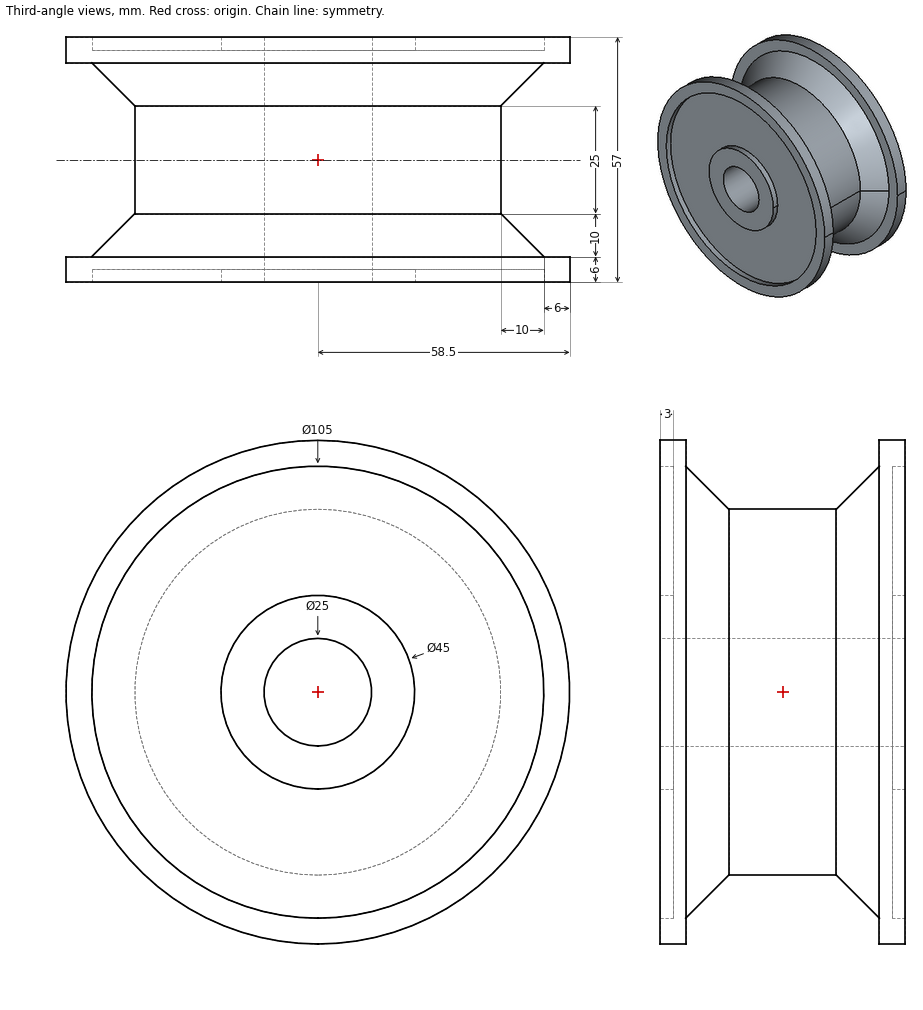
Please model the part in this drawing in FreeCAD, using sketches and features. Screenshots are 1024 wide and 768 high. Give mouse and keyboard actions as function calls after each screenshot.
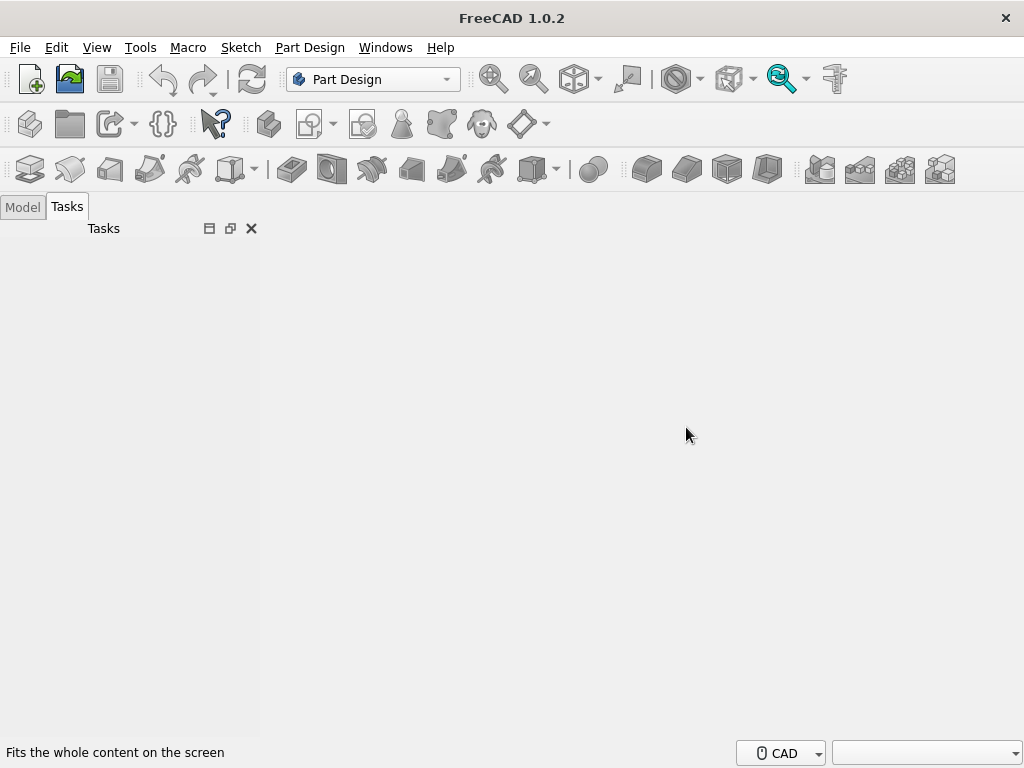
click(30, 80)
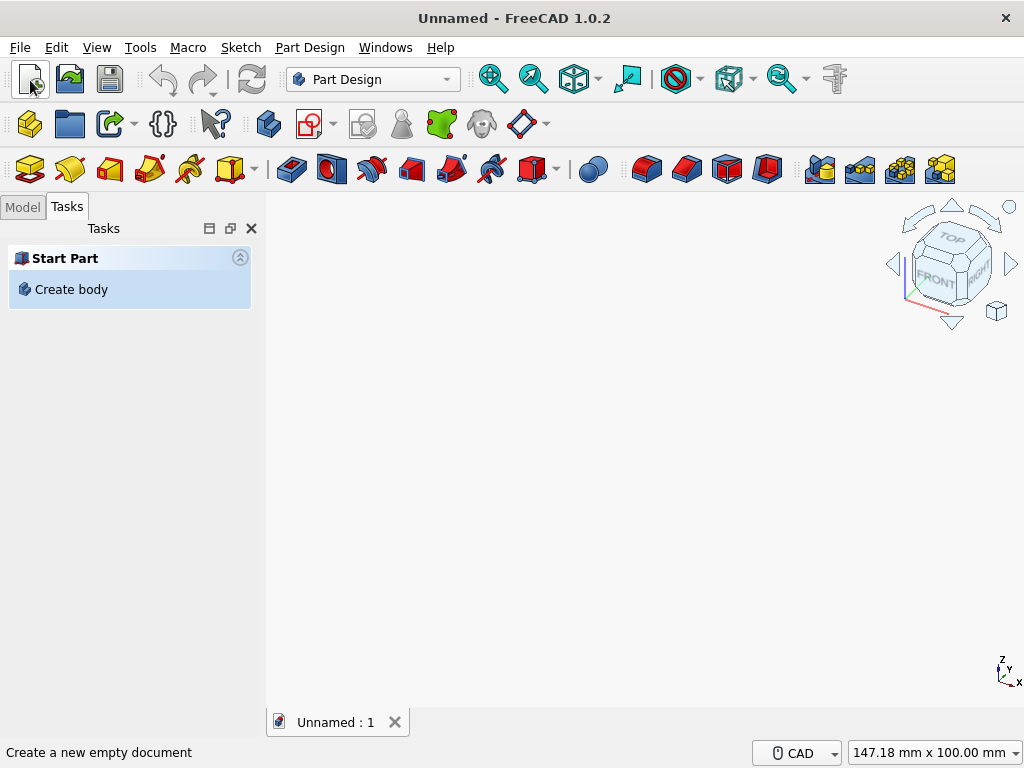
click(310, 124)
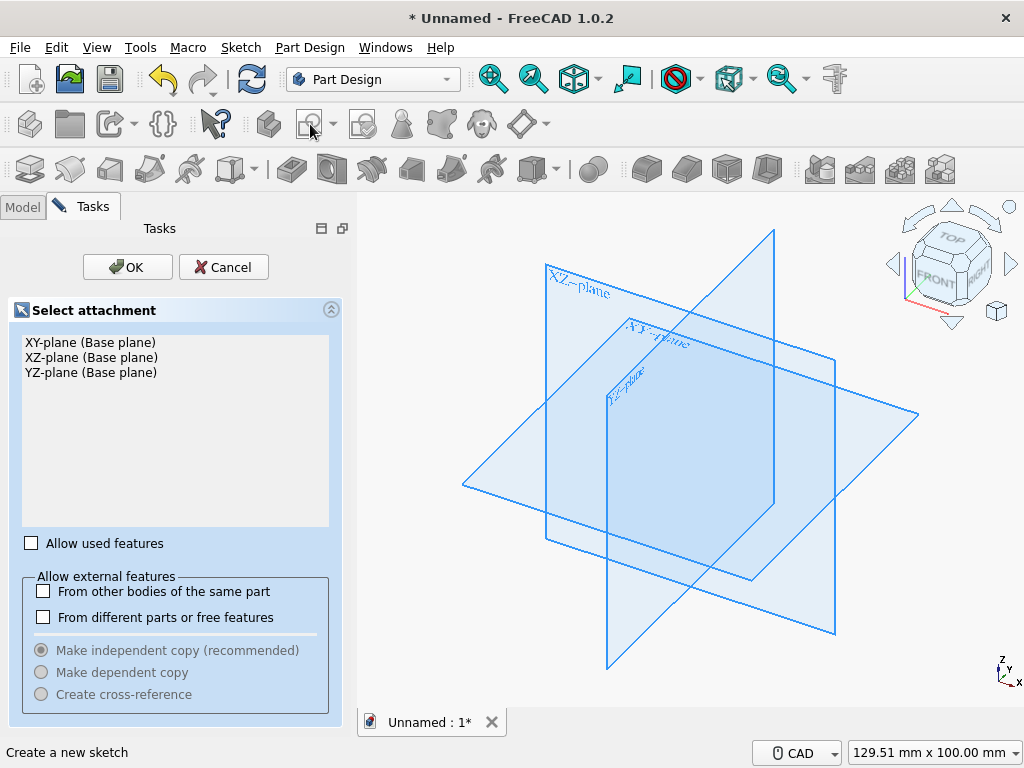
click(82, 342)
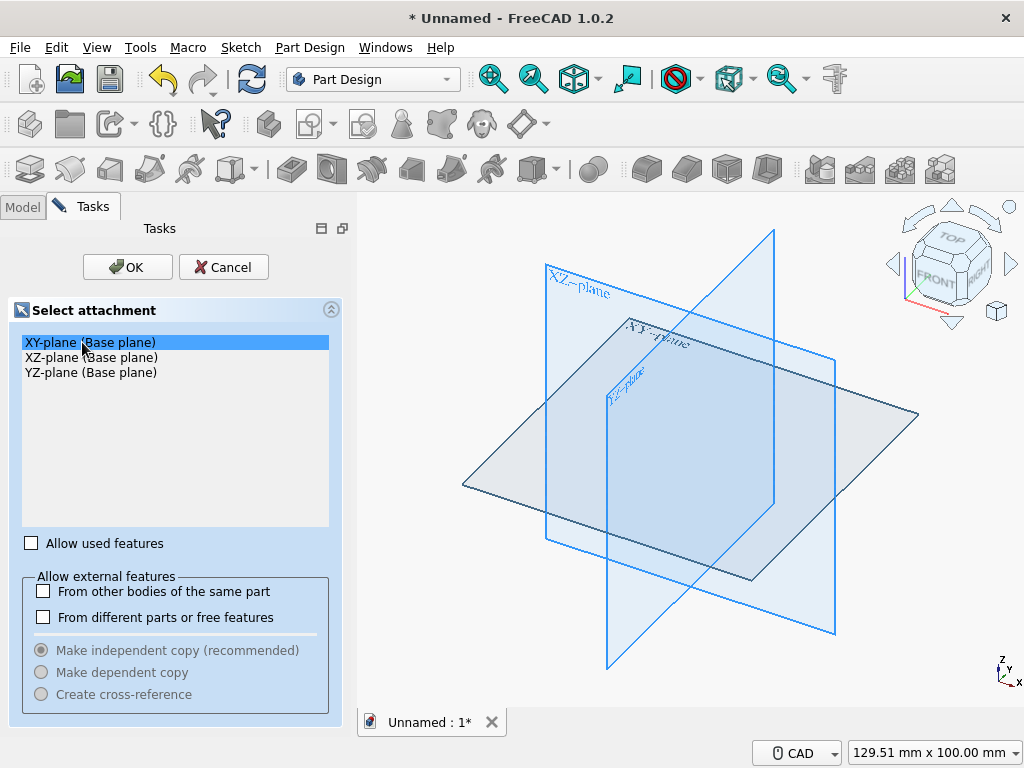
click(128, 267)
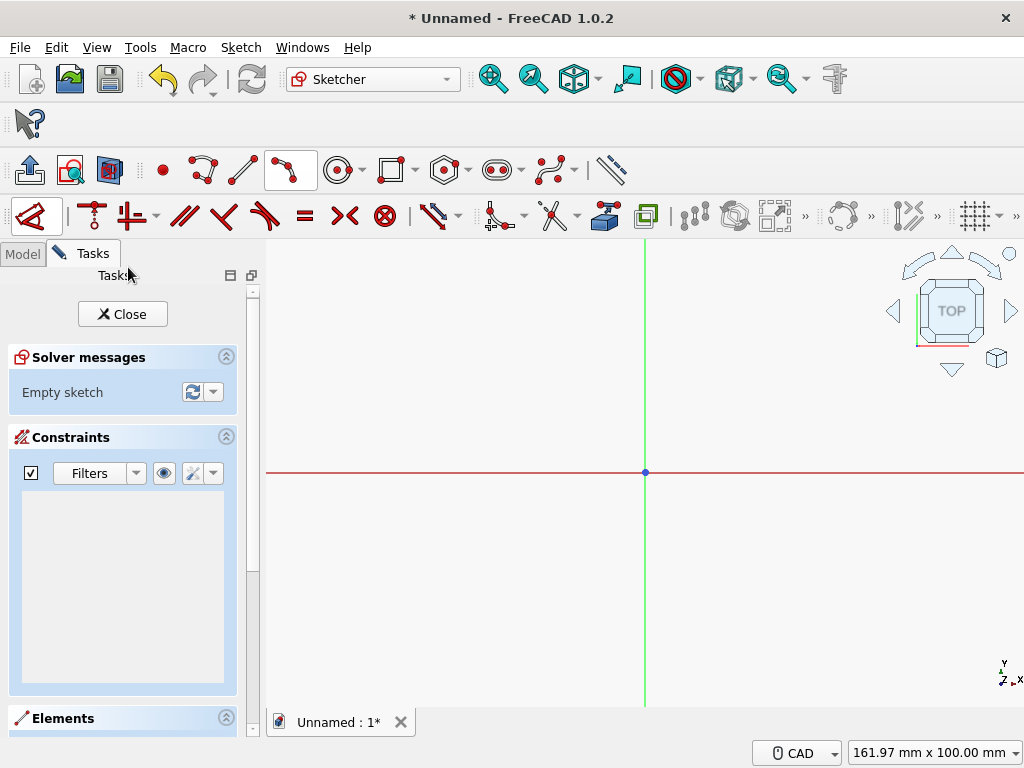
scroll(294, 473, down, 1)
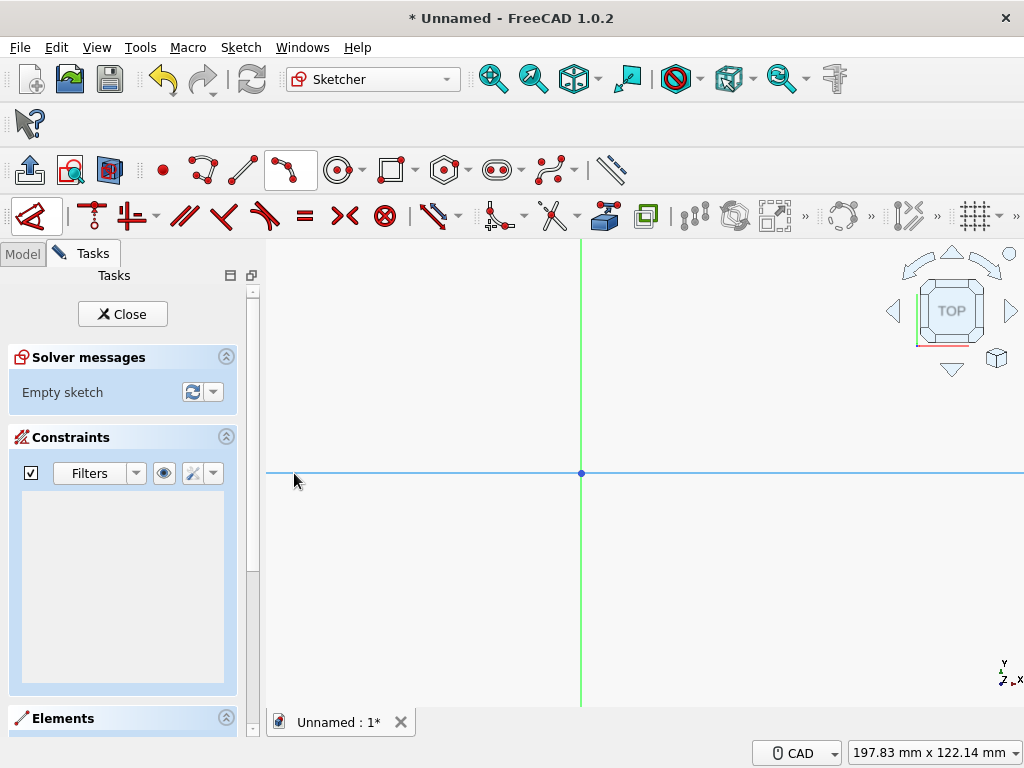
click(204, 170)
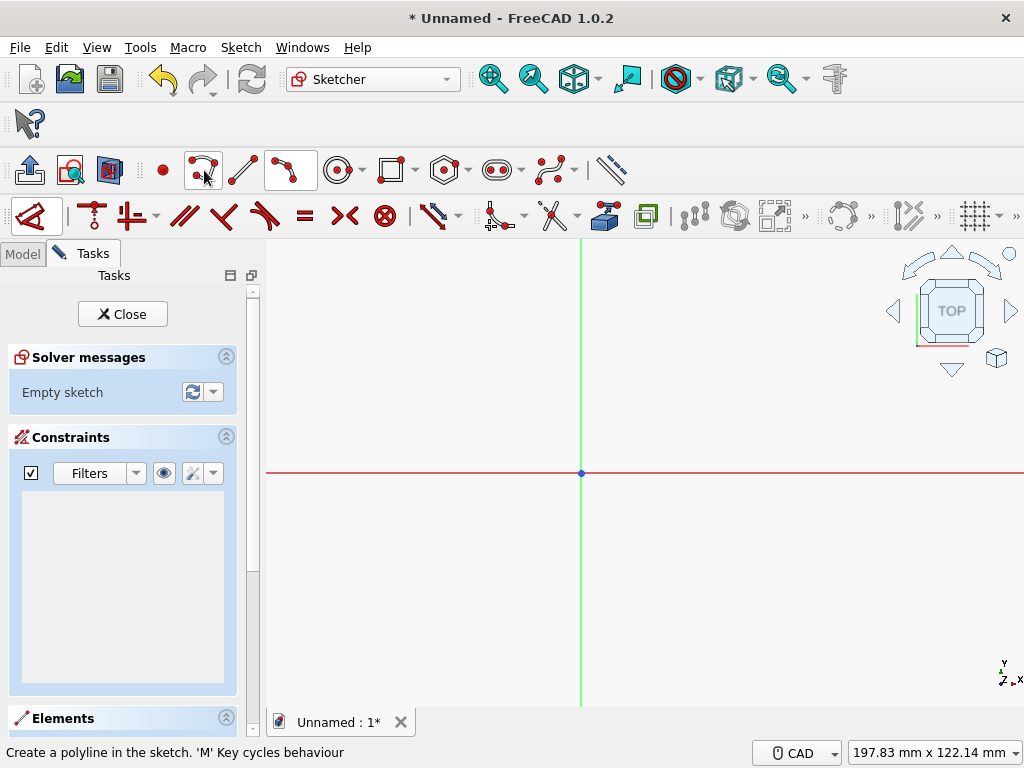
click(581, 364)
click(590, 582)
click(806, 582)
click(806, 559)
click(783, 559)
click(744, 521)
click(744, 425)
click(783, 387)
click(806, 387)
click(806, 364)
click(581, 365)
key(Escape)
key(Escape)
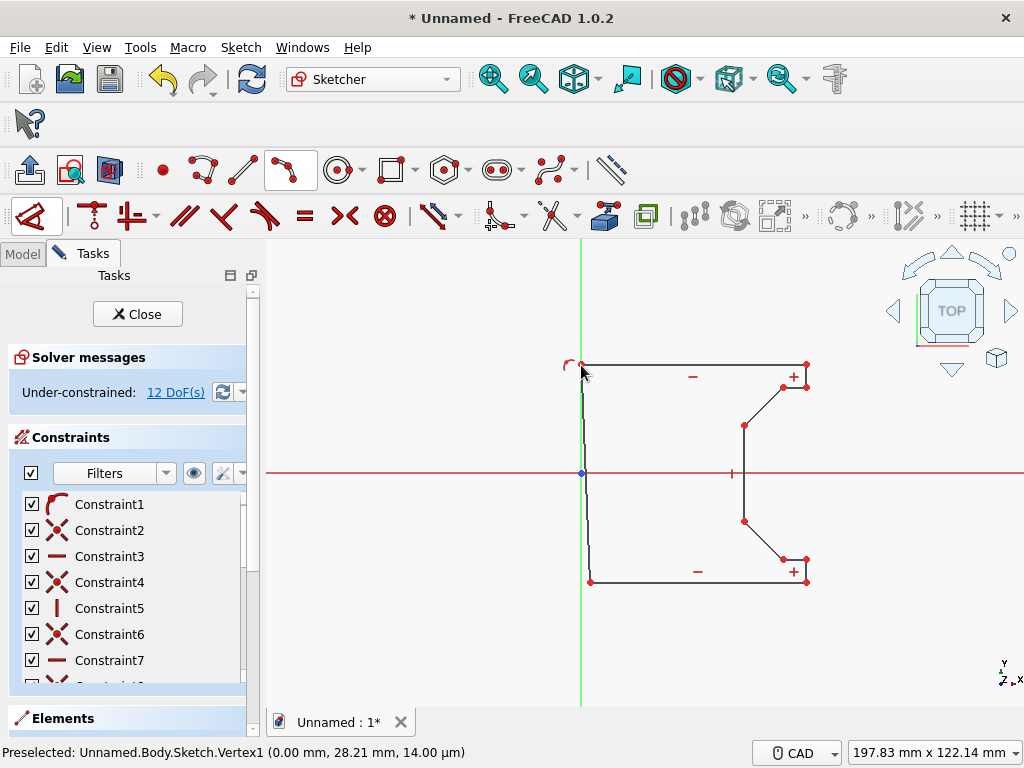
click(584, 430)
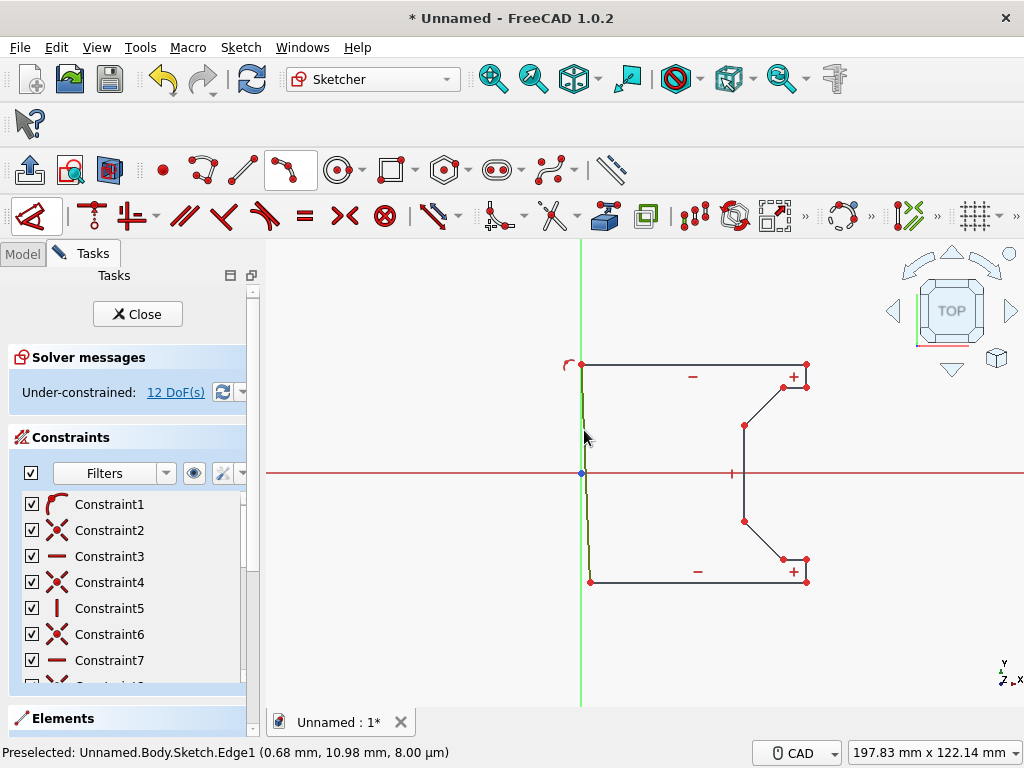
key(v)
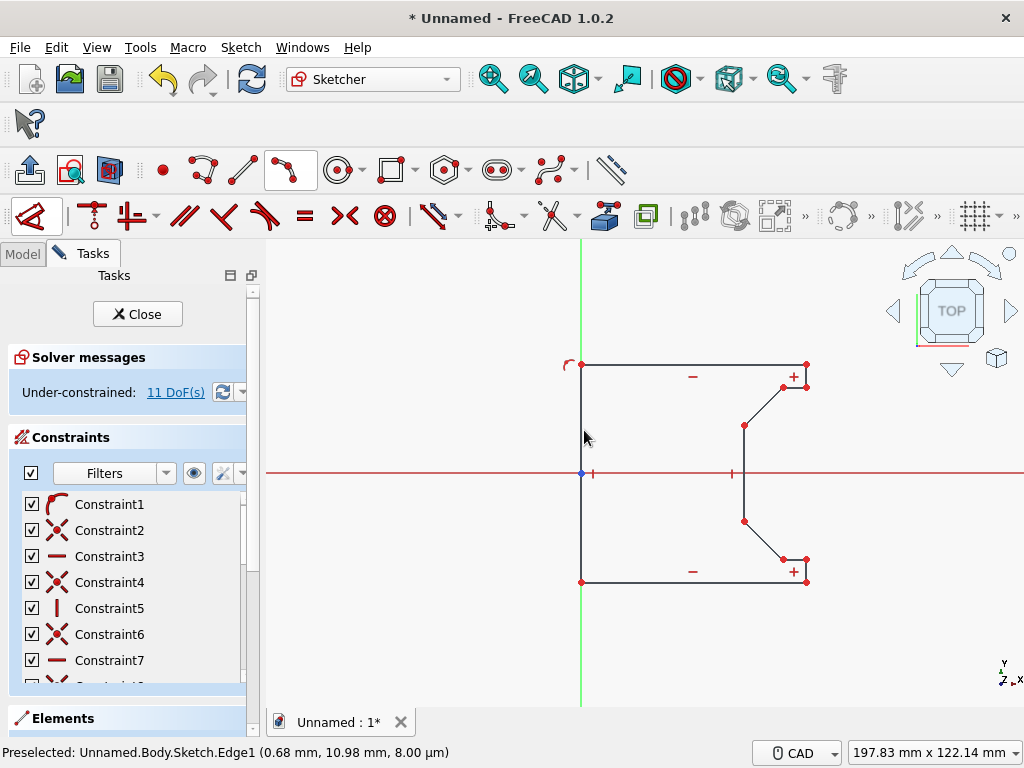
click(783, 560)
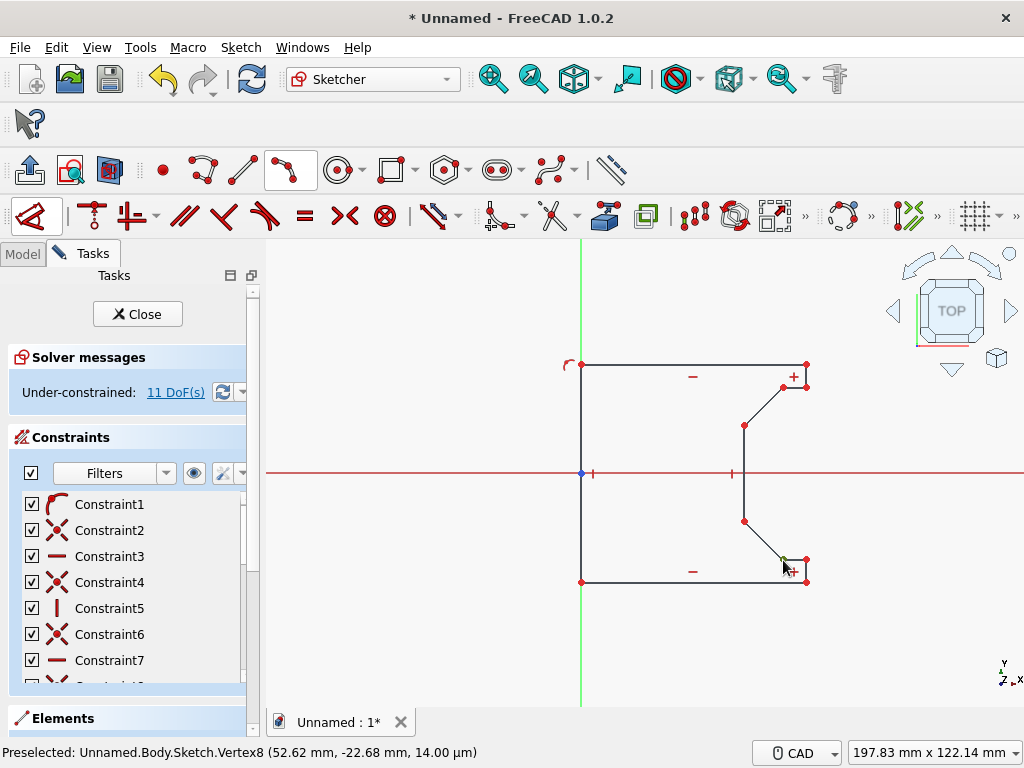
click(783, 388)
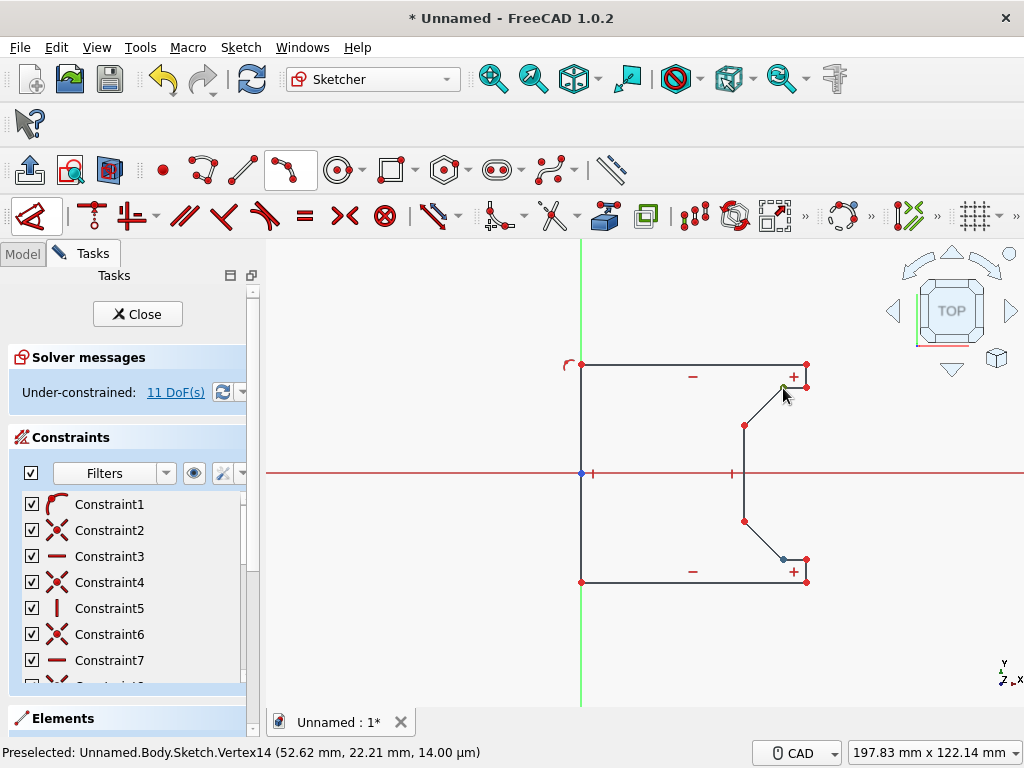
click(334, 473)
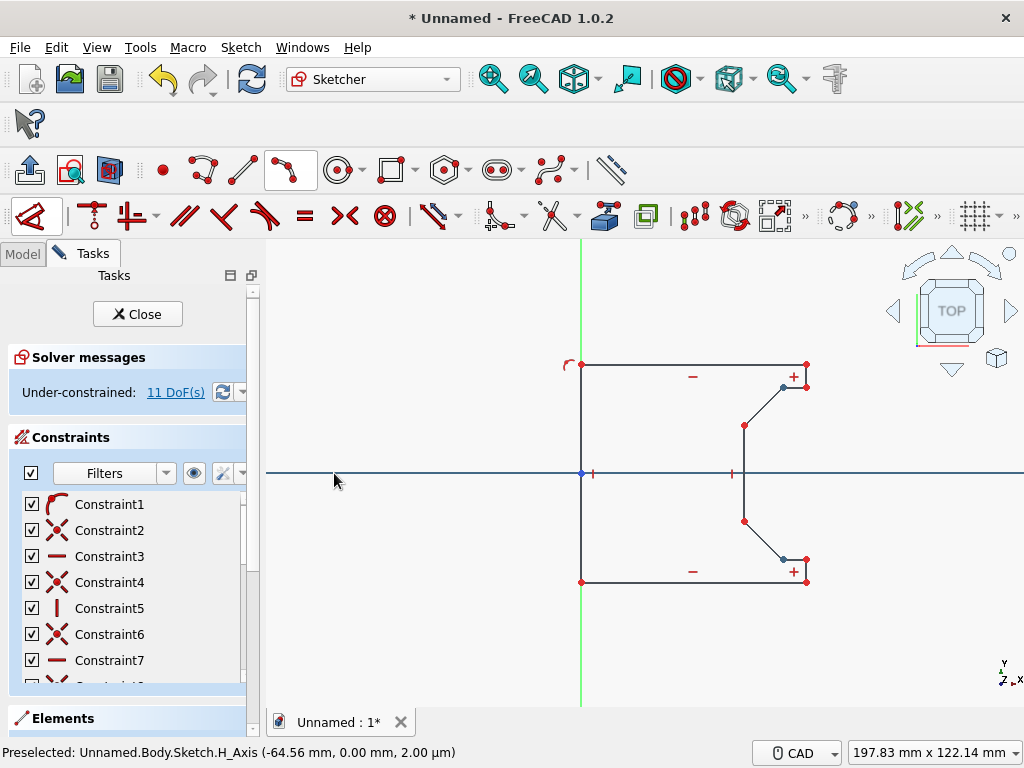
click(346, 216)